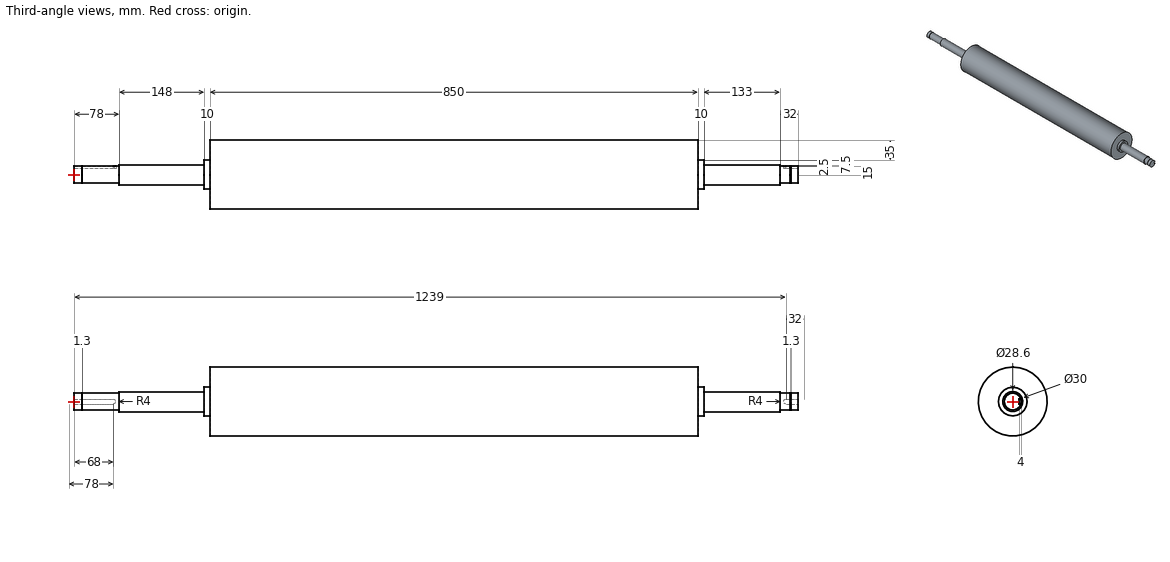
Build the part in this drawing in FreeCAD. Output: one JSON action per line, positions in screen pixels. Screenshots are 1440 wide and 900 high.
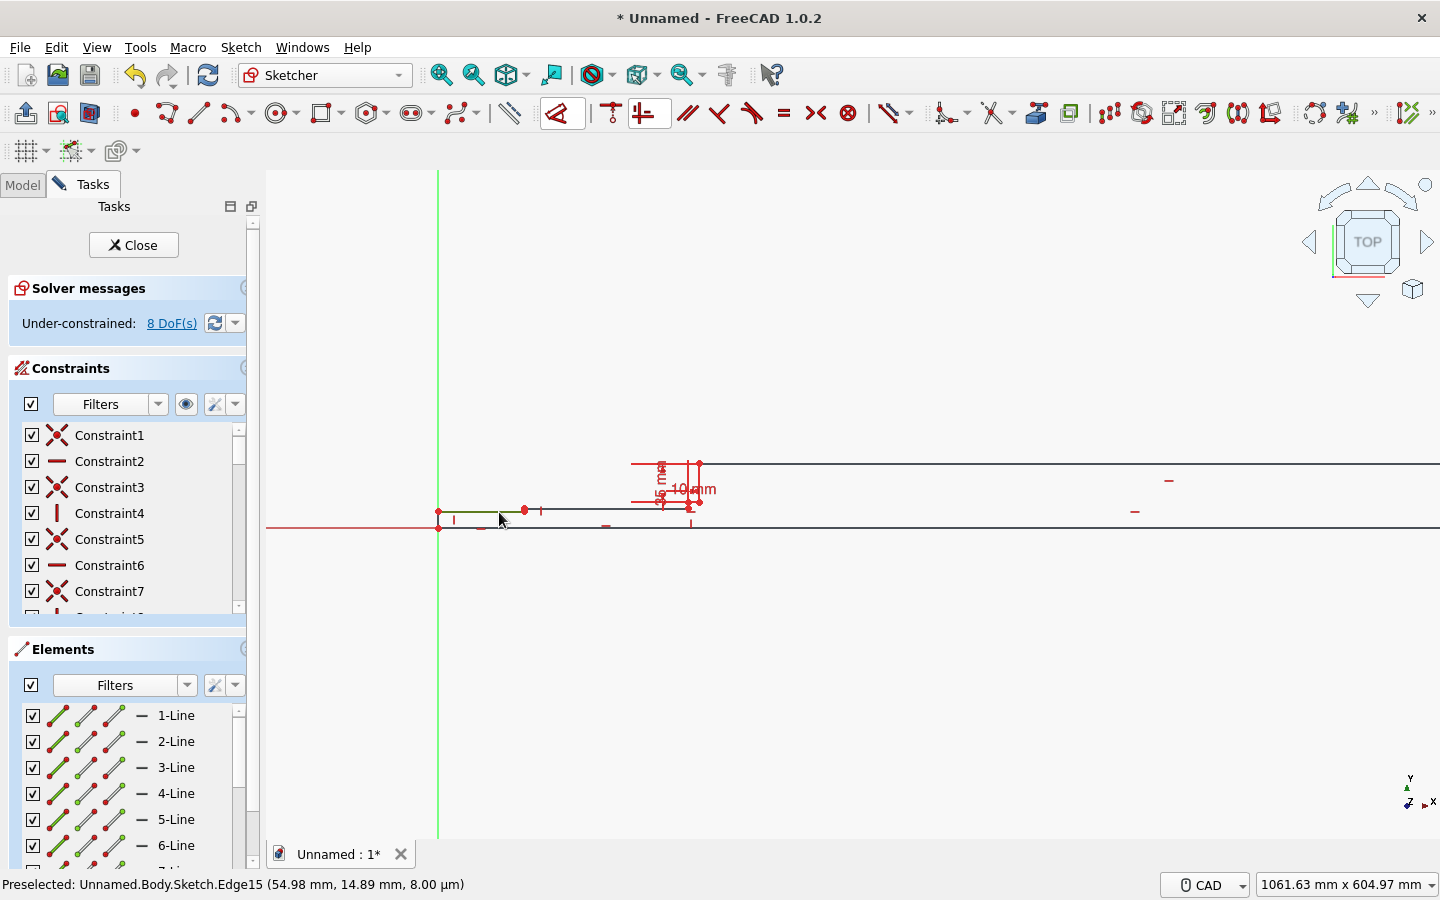
{"action": "key", "text": "l"}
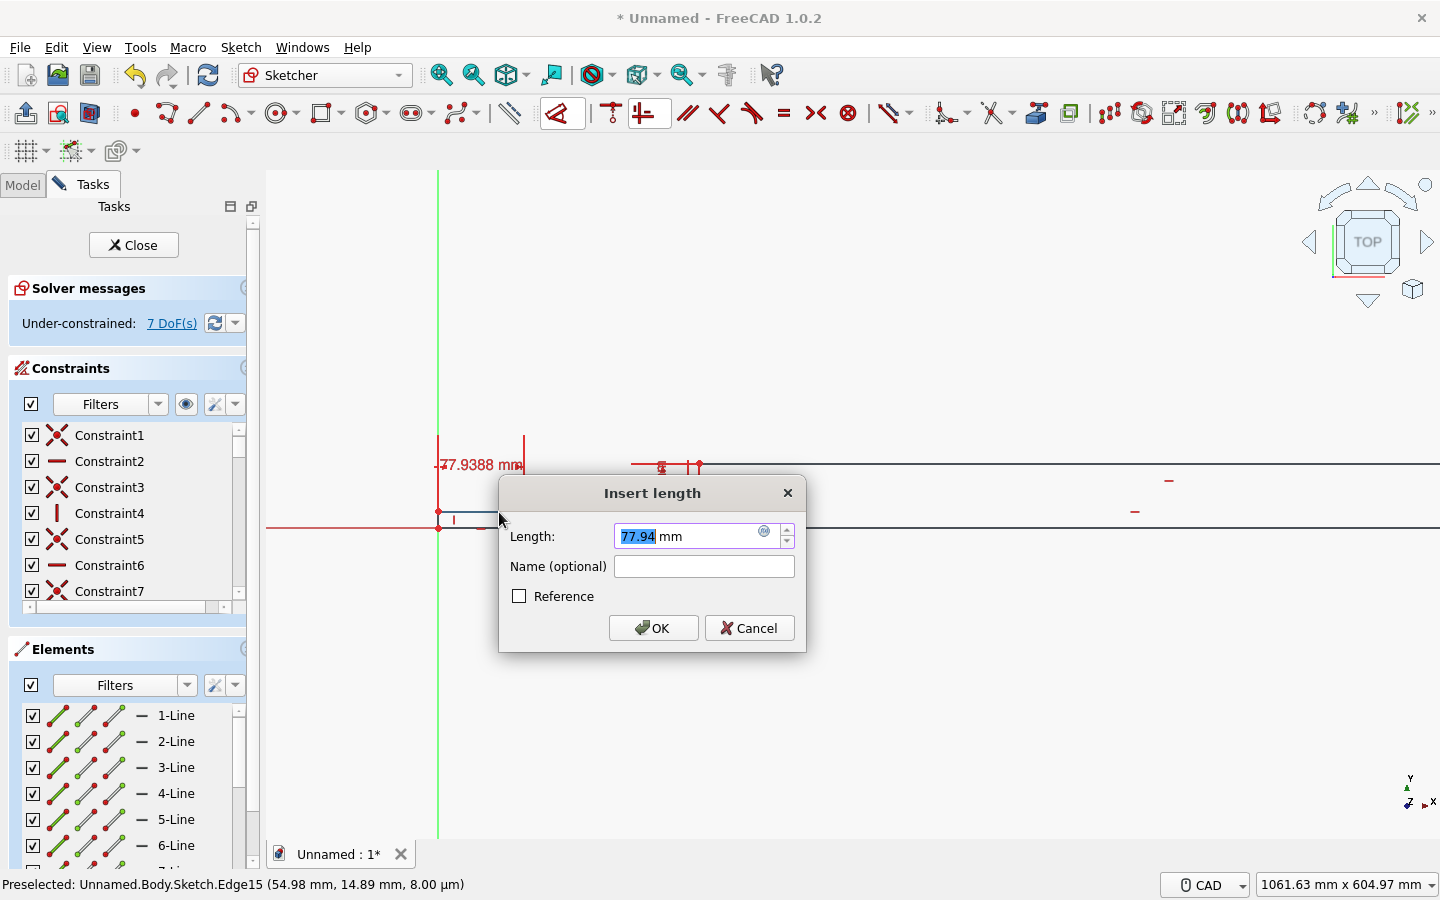
{"action": "type", "text": "78"}
{"action": "key", "text": "Return"}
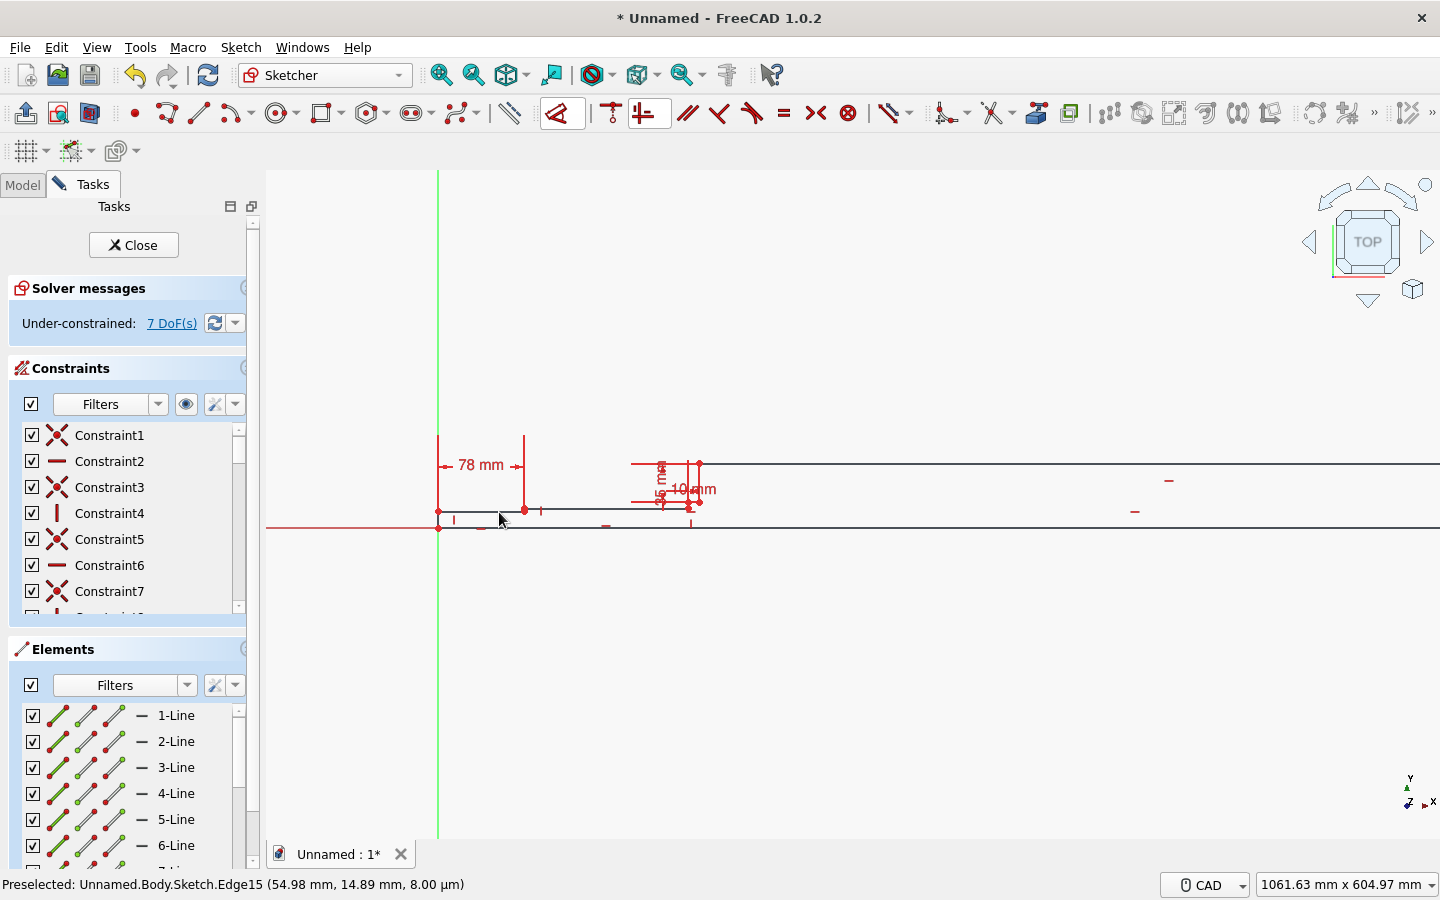
{"action": "scroll", "coordinate": [438, 520], "scroll_direction": "up", "scroll_amount": 5}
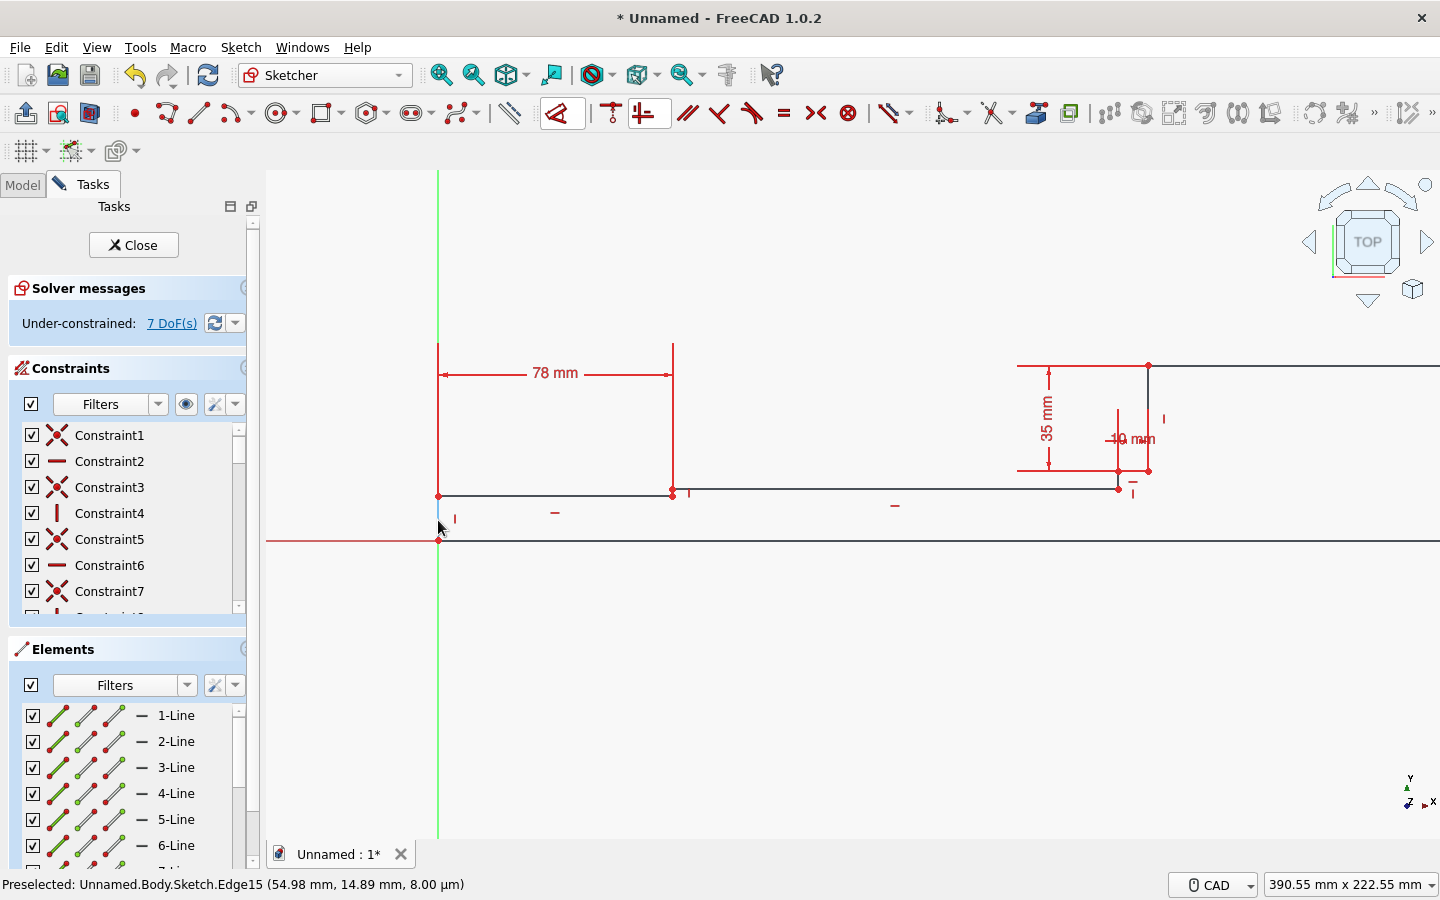
{"action": "left_click", "coordinate": [438, 519]}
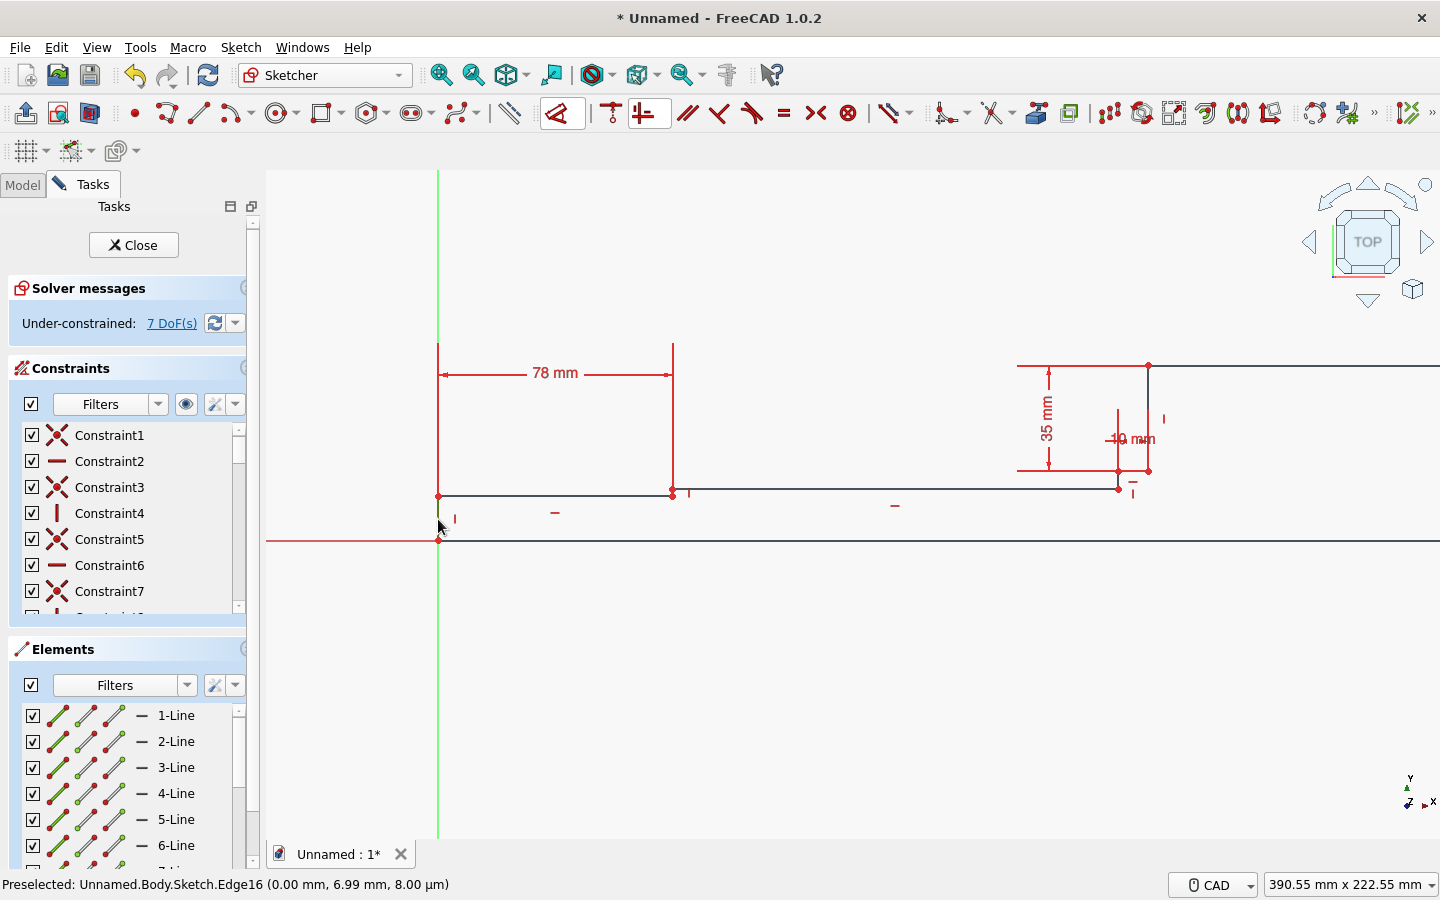
{"action": "key", "text": "i"}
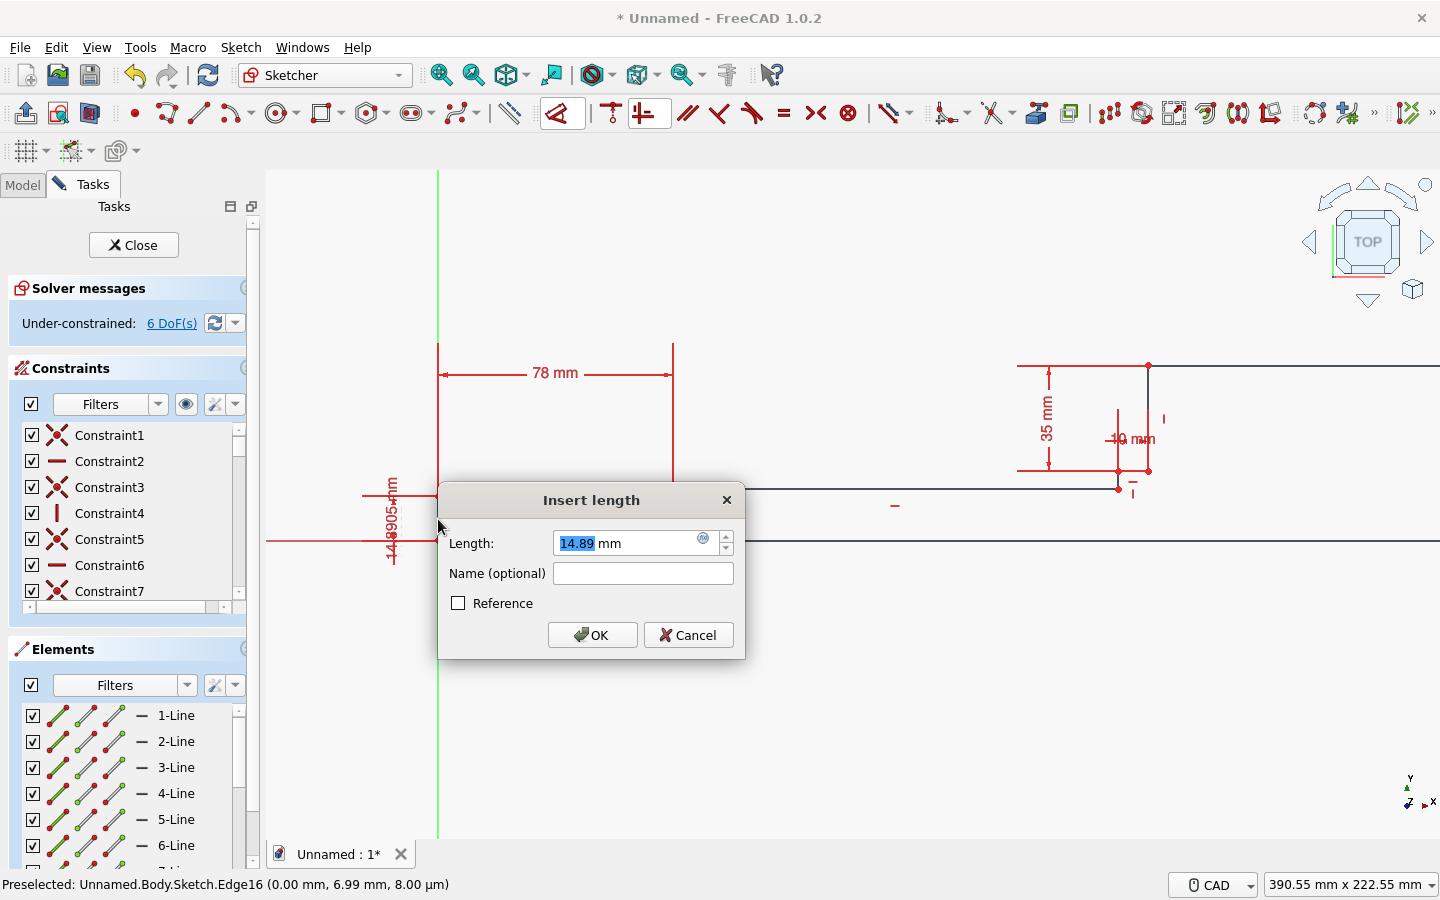
{"action": "type", "text": "15"}
{"action": "key", "text": "Return"}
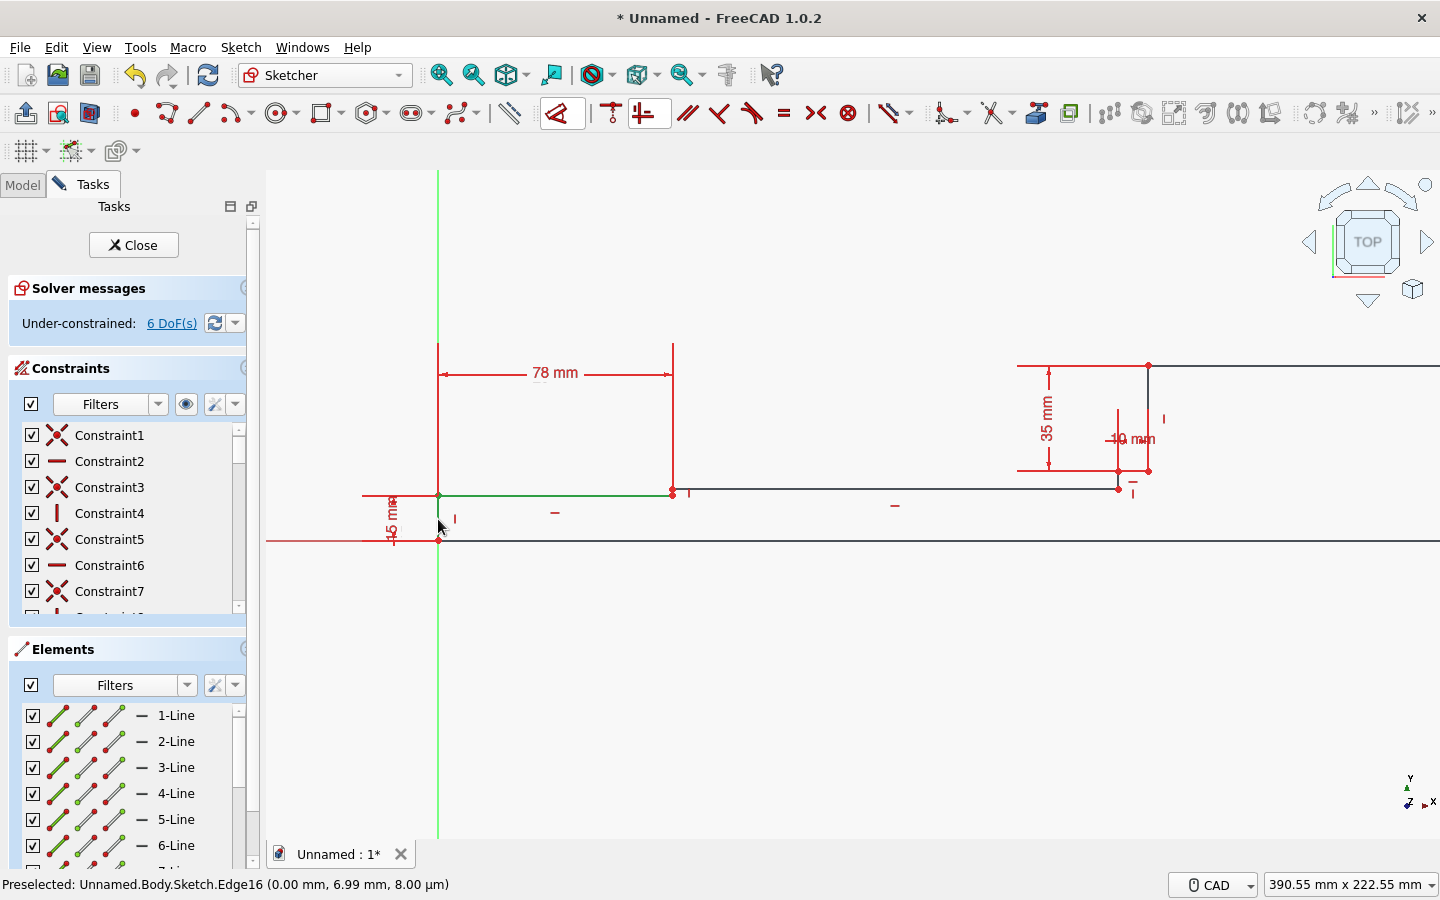
{"action": "scroll", "coordinate": [478, 515], "scroll_direction": "down", "scroll_amount": 9}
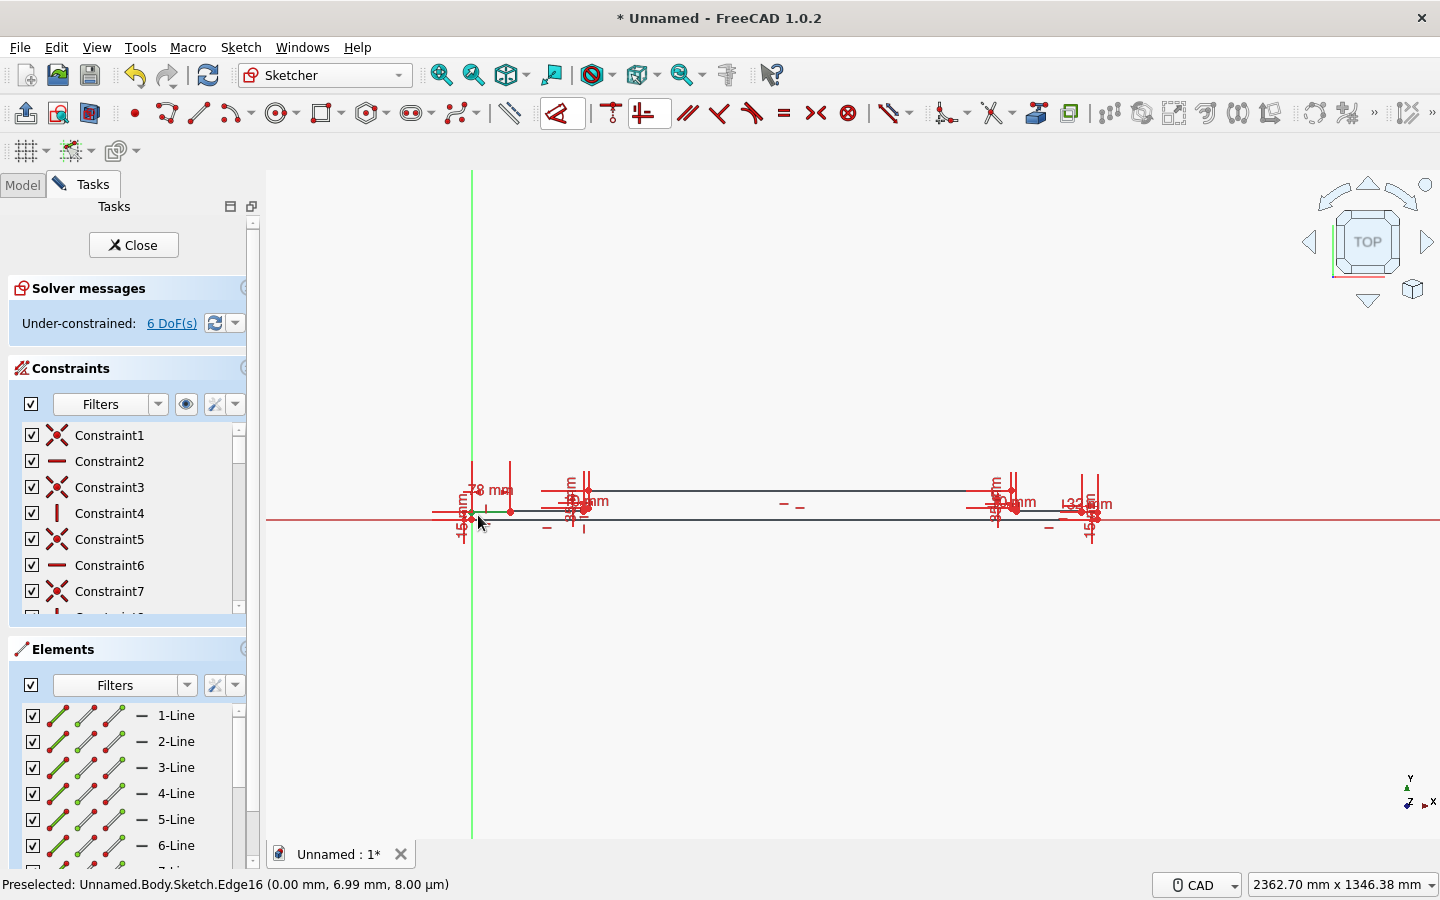
{"action": "scroll", "coordinate": [1082, 512], "scroll_direction": "up", "scroll_amount": 18}